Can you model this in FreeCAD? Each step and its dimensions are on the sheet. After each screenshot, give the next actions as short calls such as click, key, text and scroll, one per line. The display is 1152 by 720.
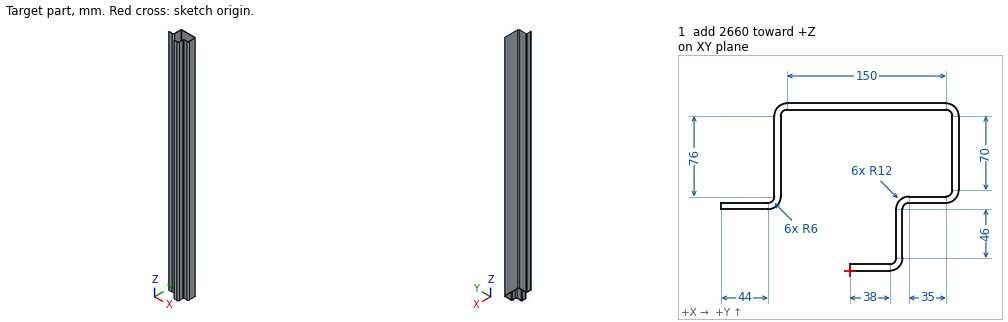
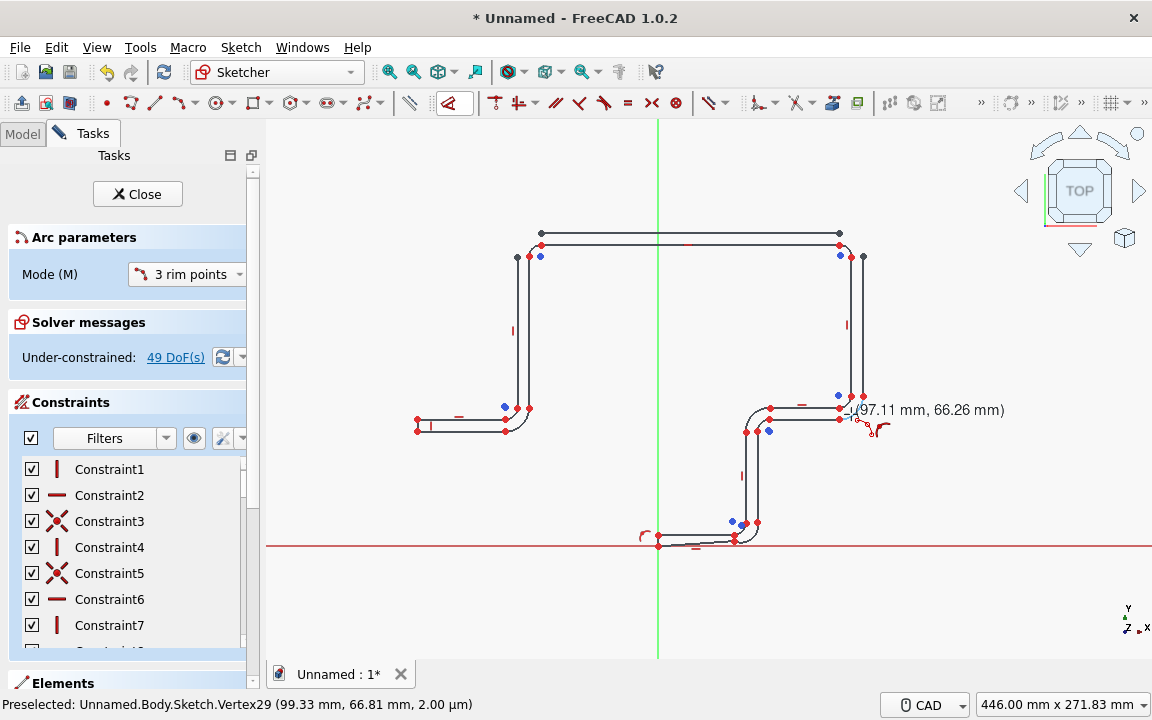
scroll(863, 256, up, 2)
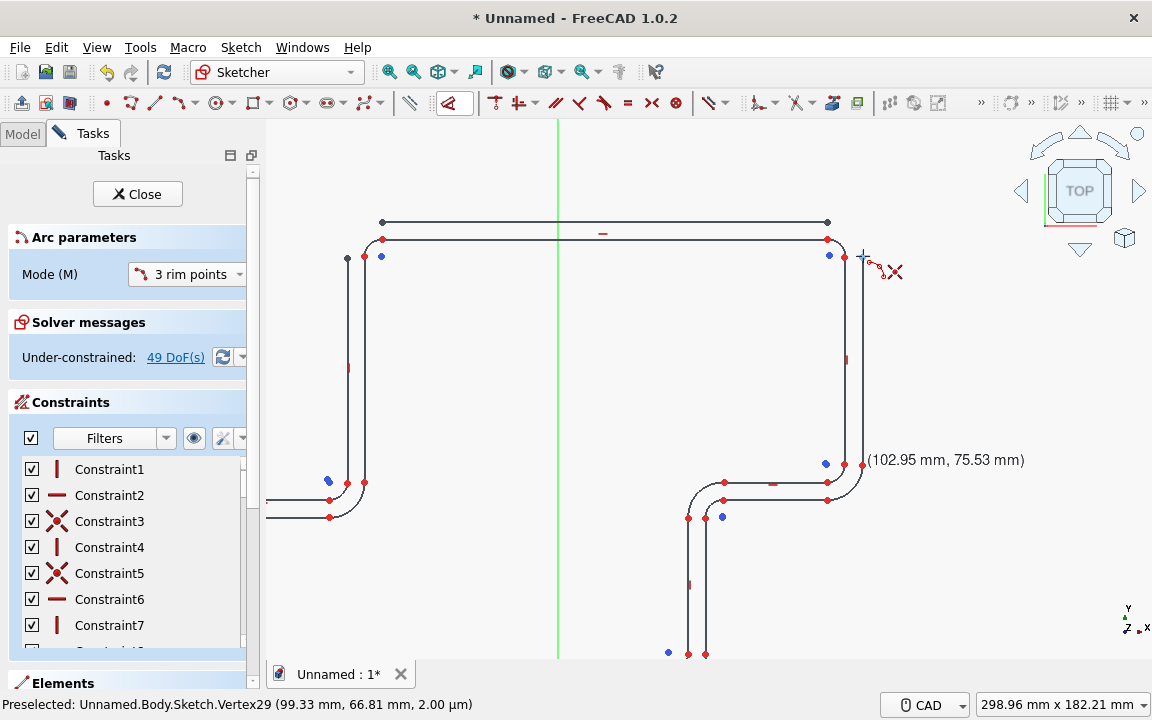
click(863, 257)
click(828, 222)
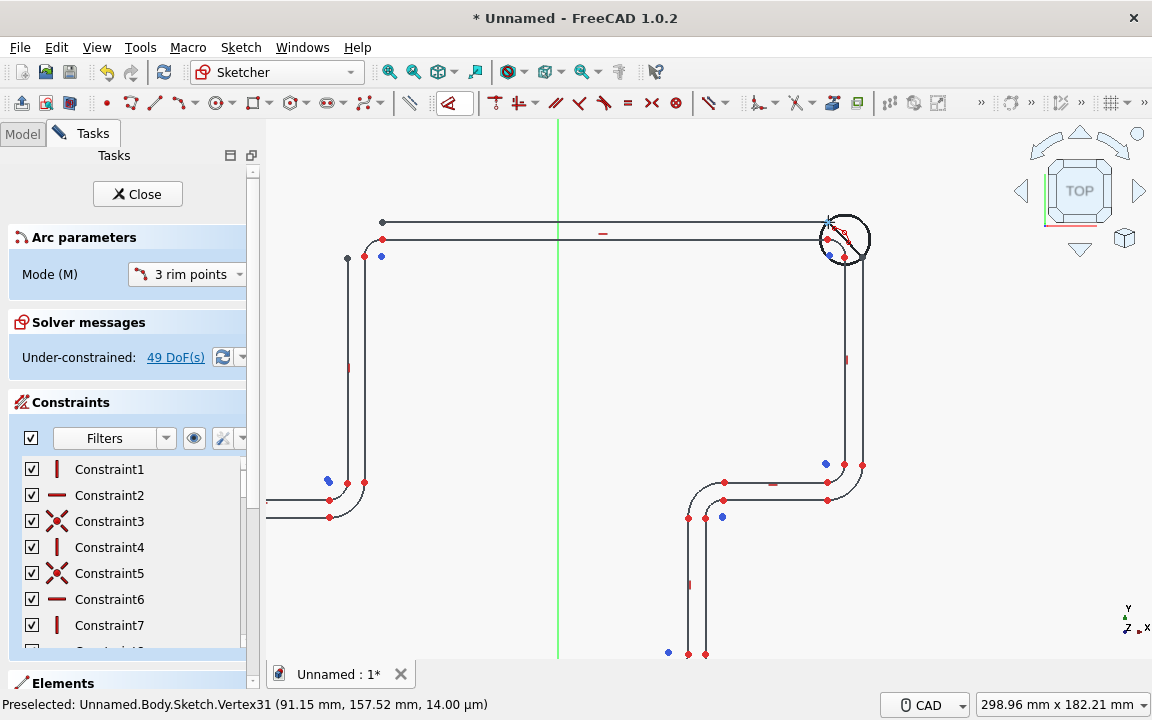
scroll(852, 231, up, 3)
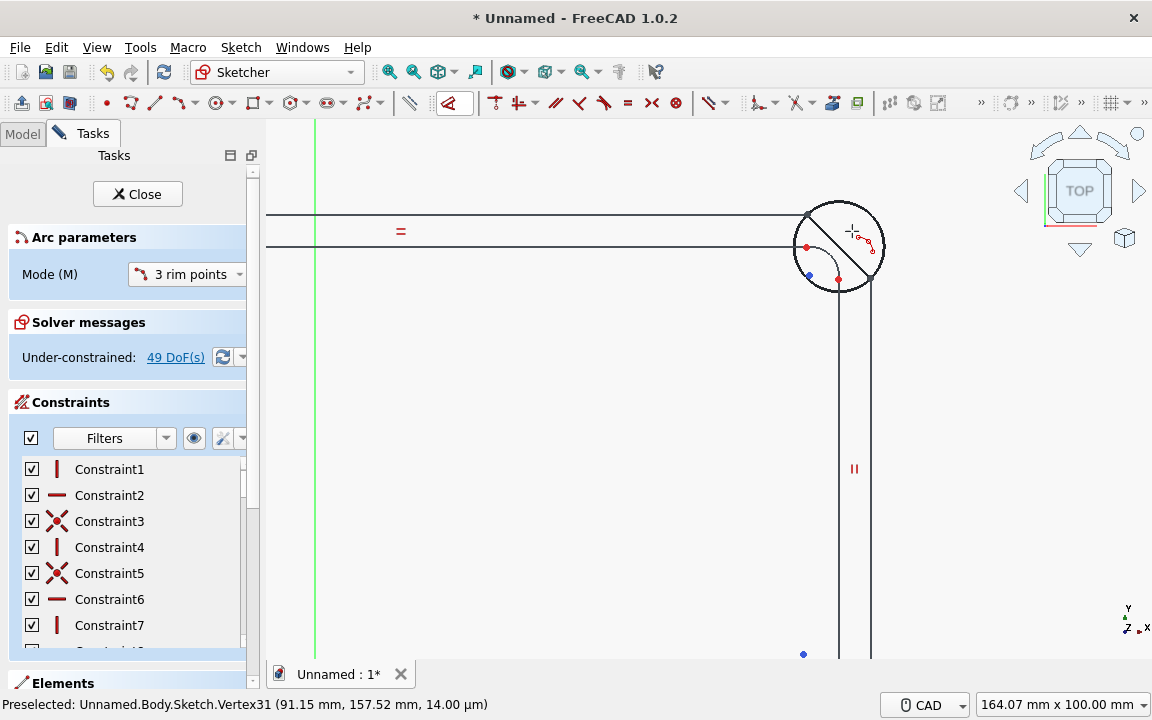
click(852, 231)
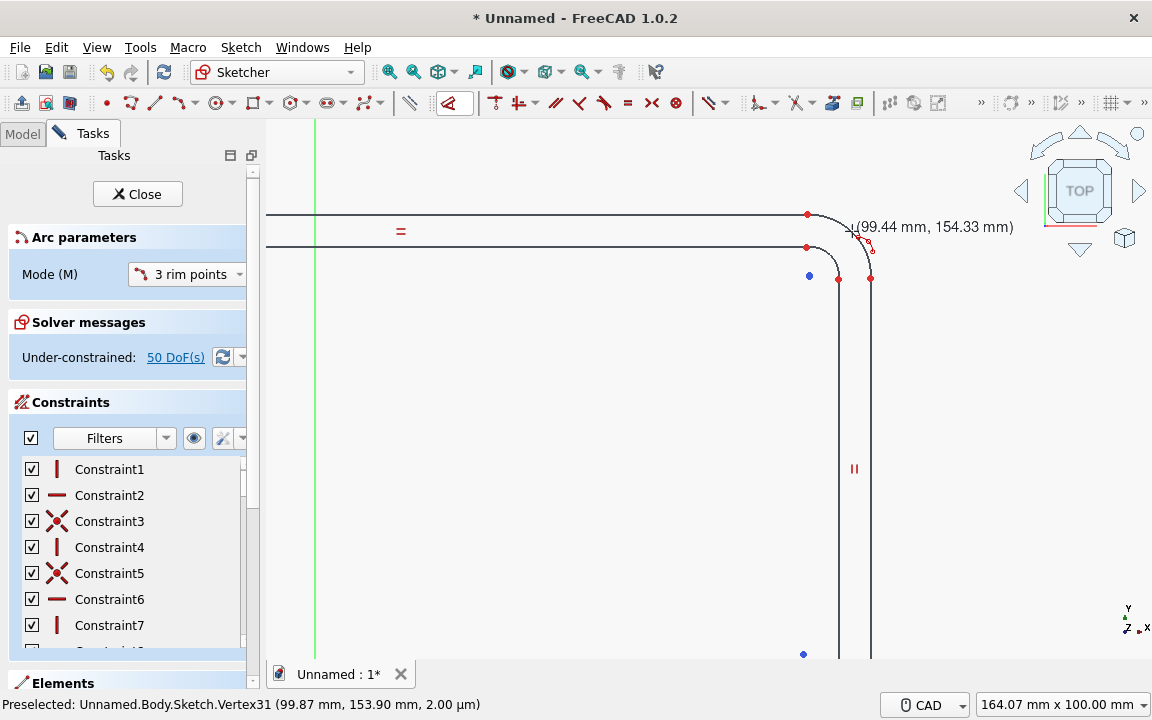
scroll(858, 244, down, 5)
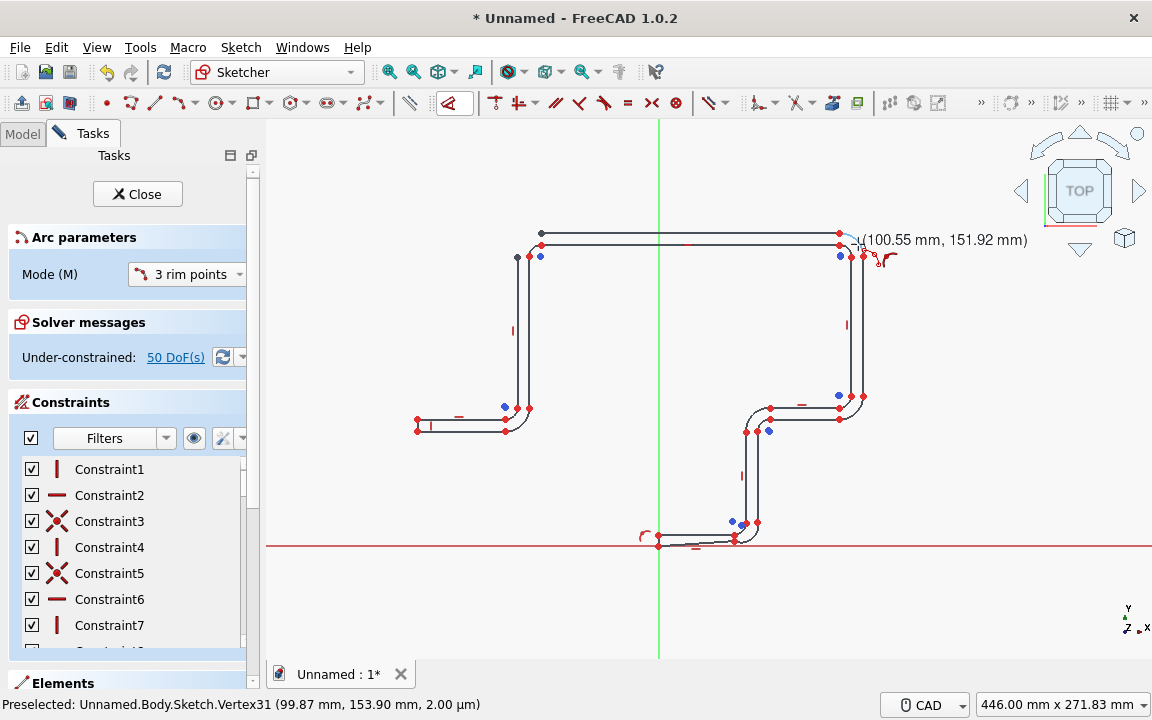
scroll(541, 232, up, 2)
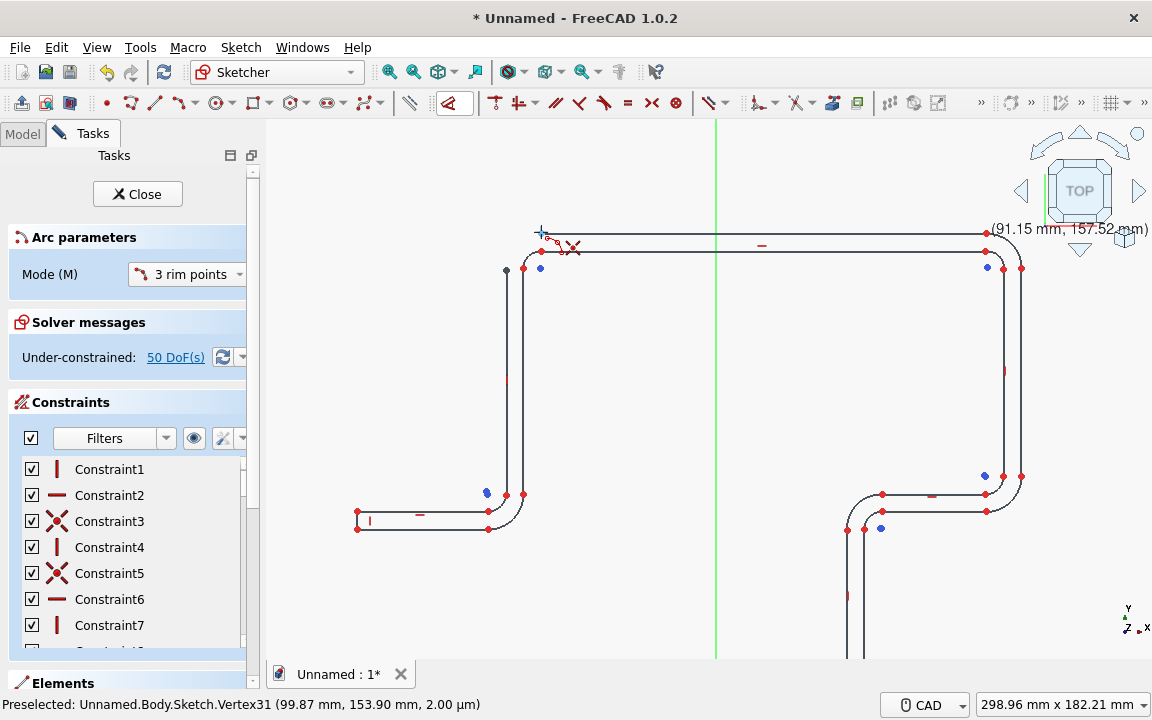
click(542, 234)
click(507, 270)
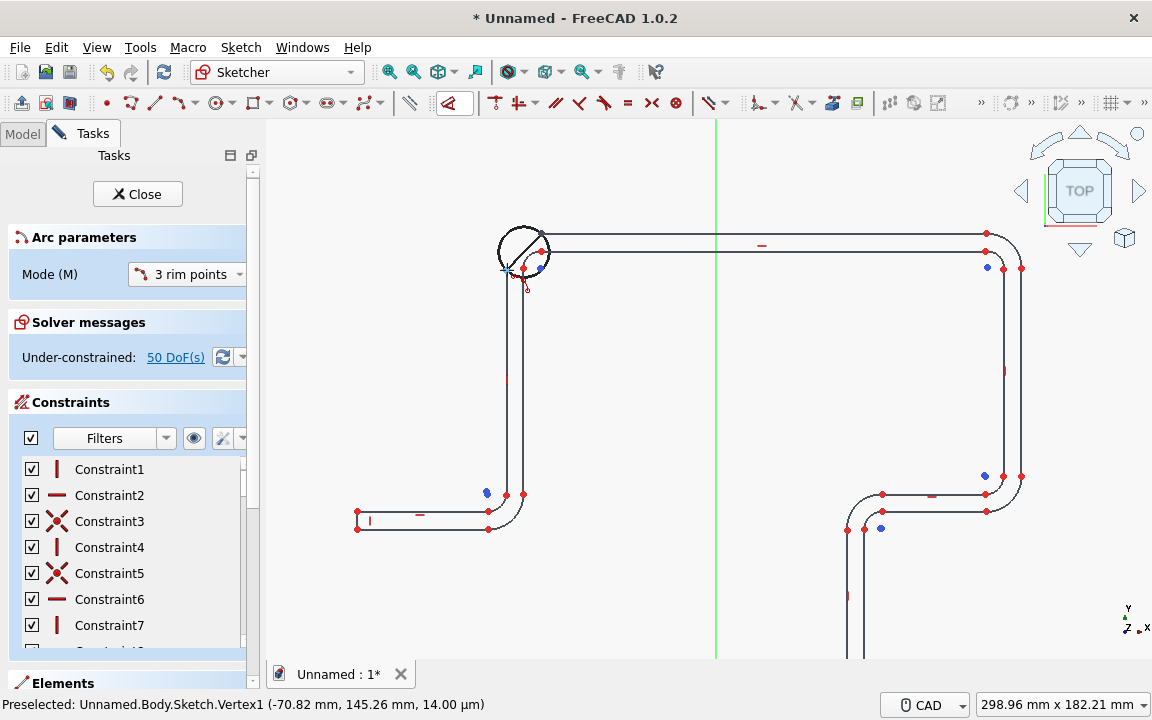
scroll(516, 243, up, 3)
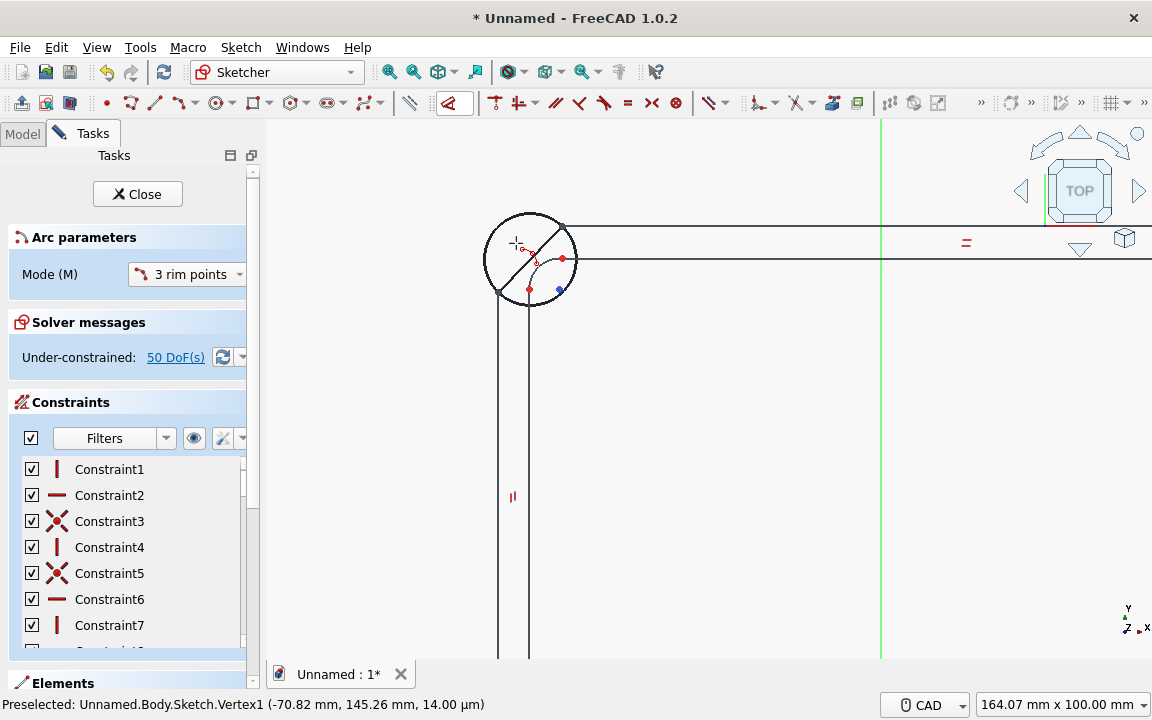
click(516, 243)
key(Escape)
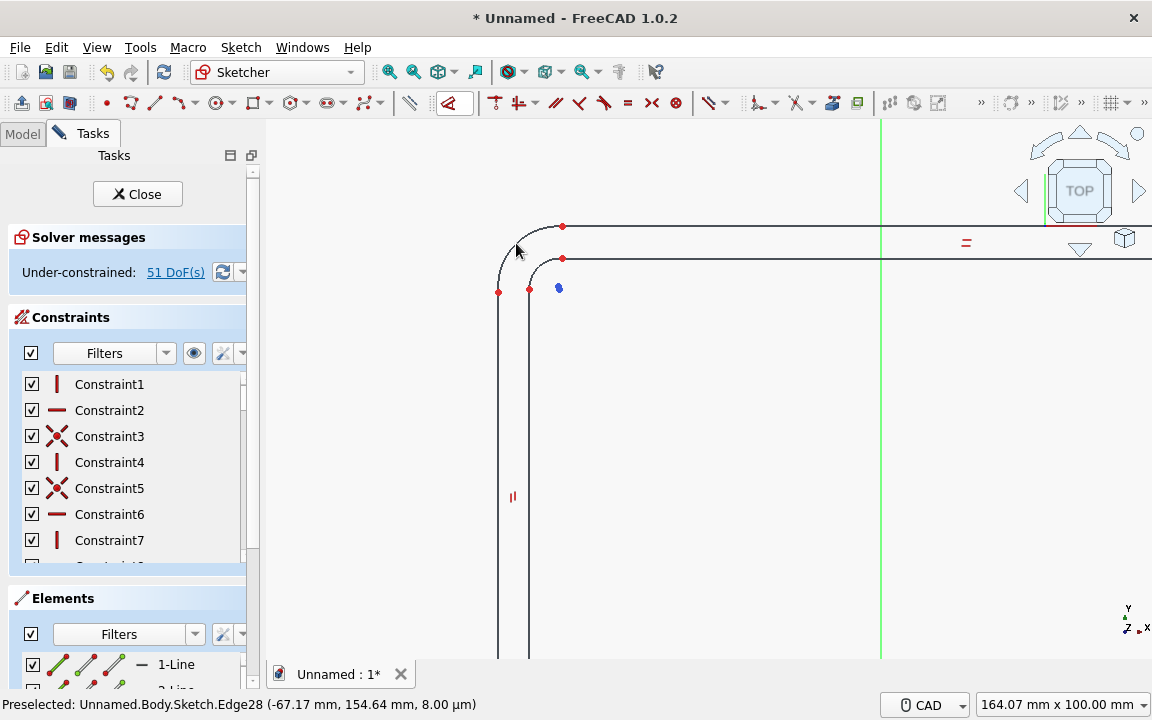
click(498, 416)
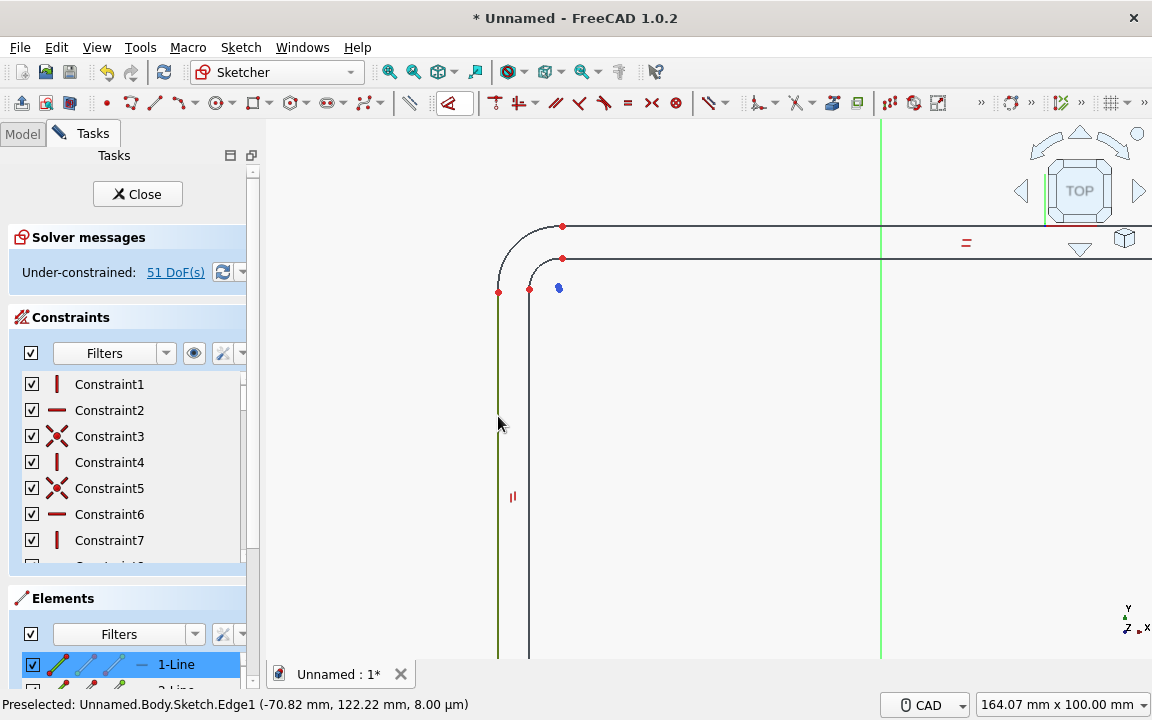
scroll(529, 237, down, 5)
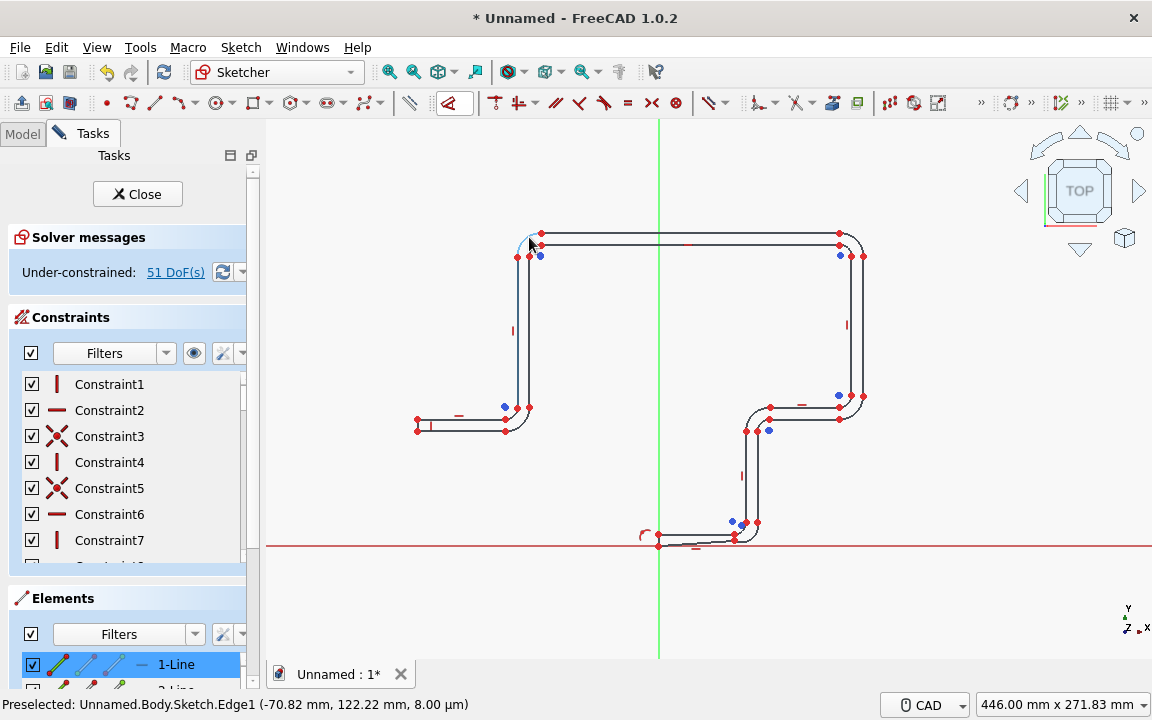
scroll(511, 418, up, 5)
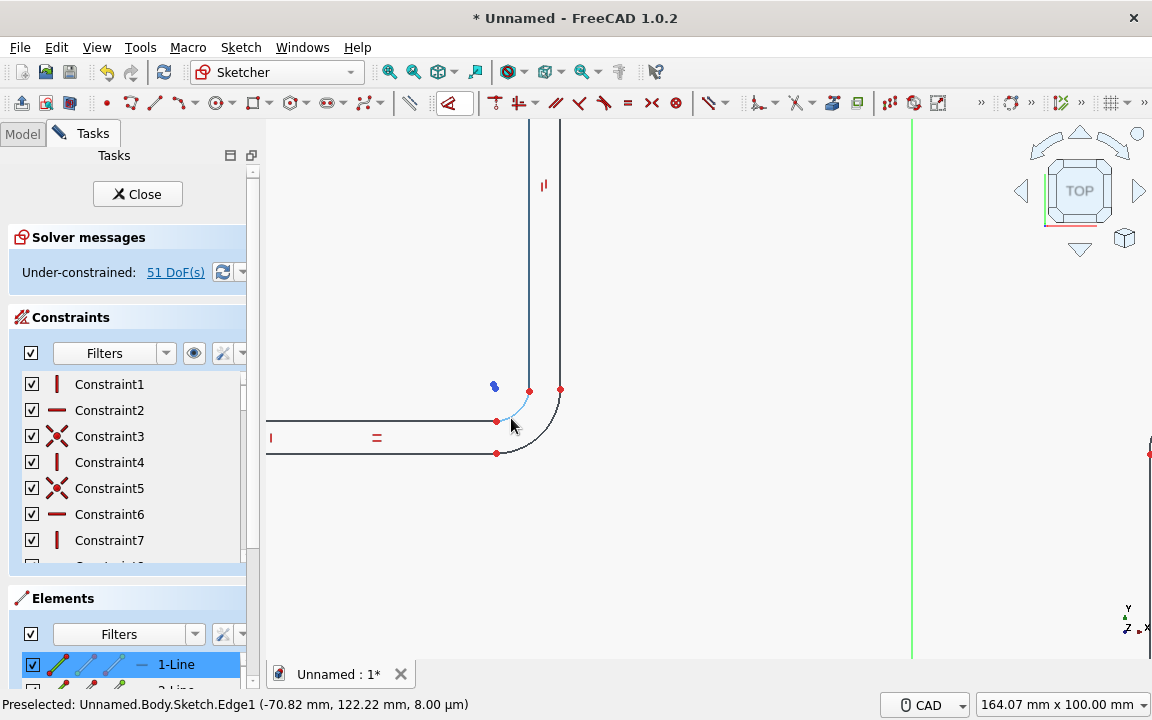
click(510, 417)